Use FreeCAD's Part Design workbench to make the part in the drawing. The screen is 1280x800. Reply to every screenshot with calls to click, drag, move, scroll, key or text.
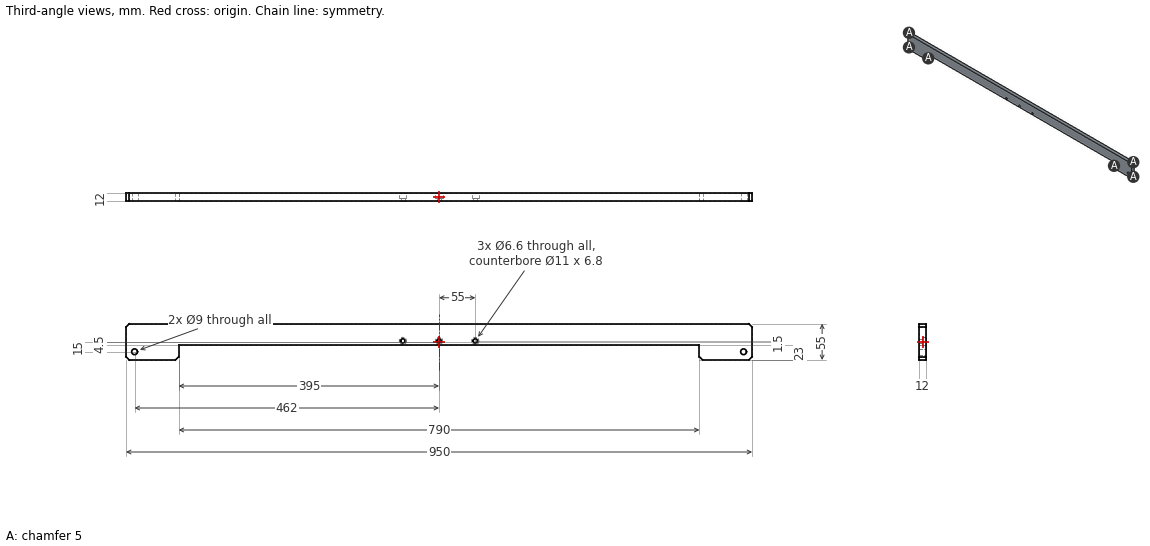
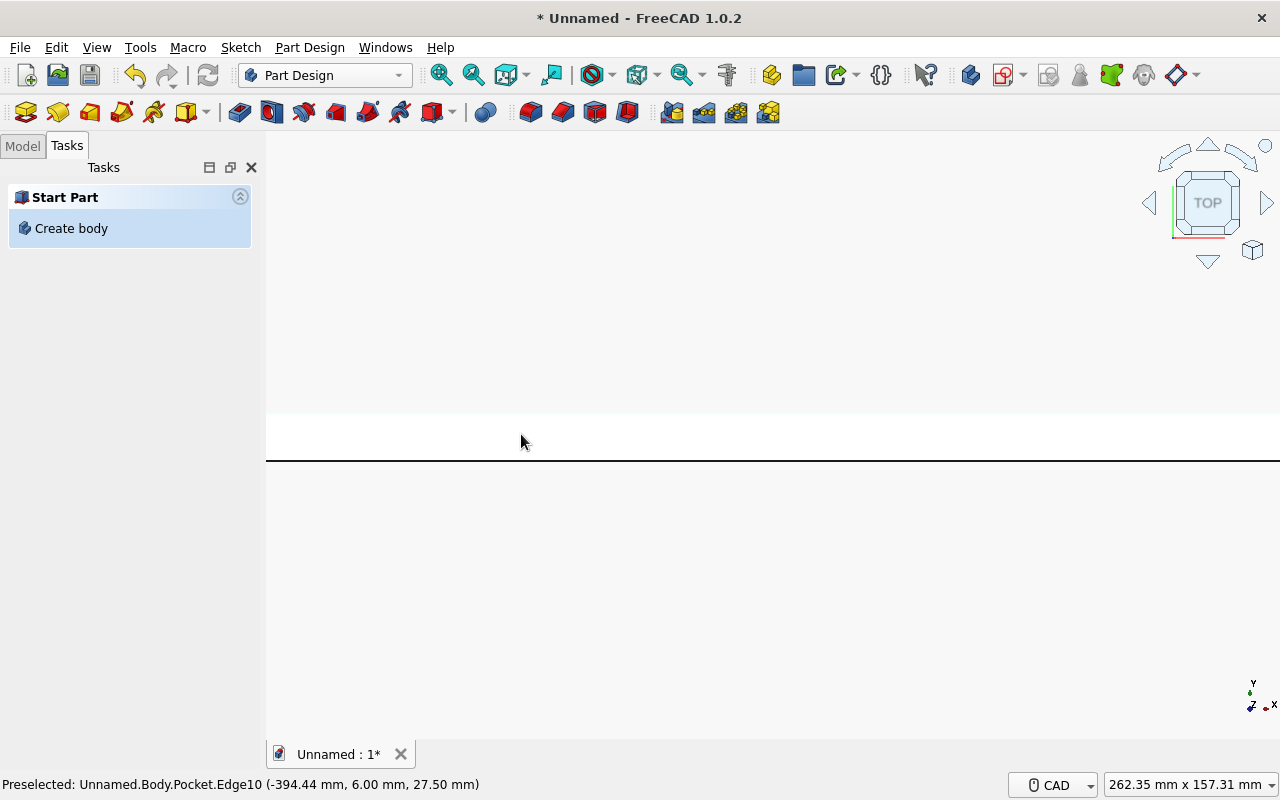
key(v)
key(f)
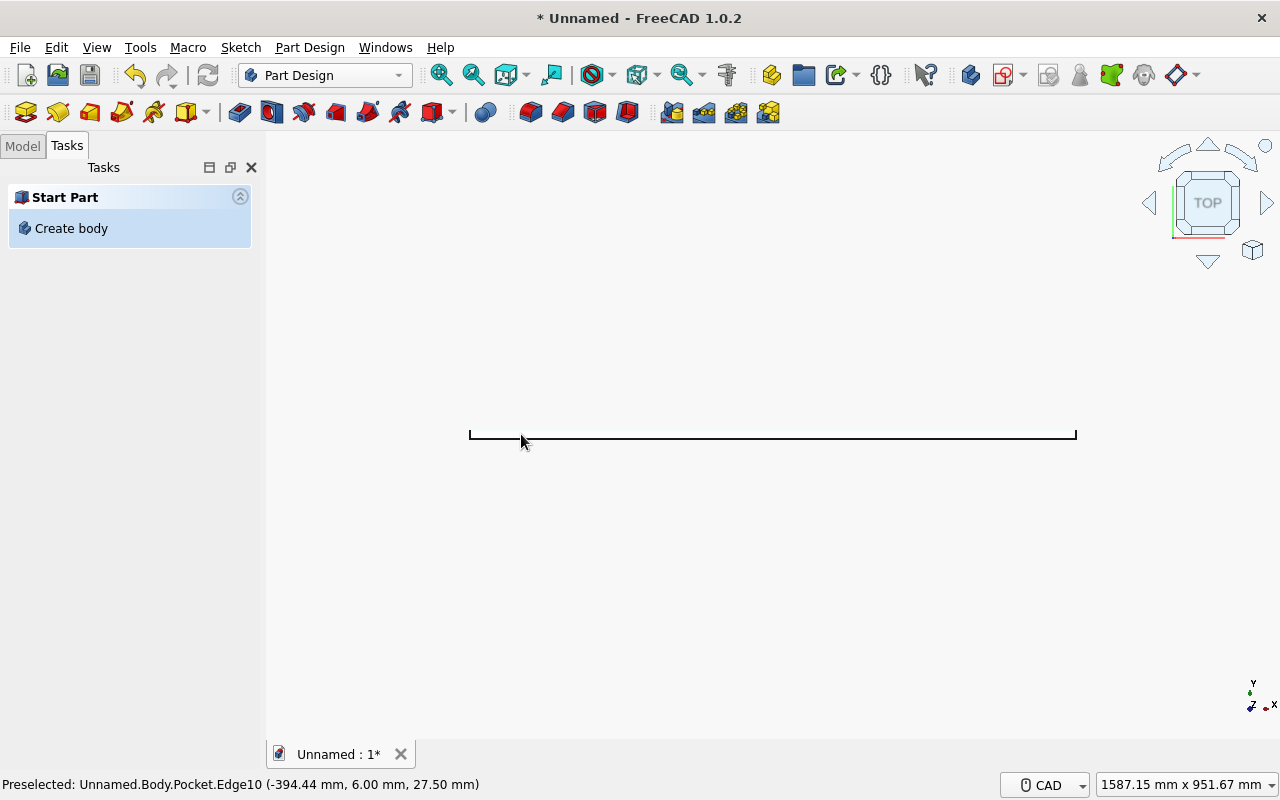
key(1)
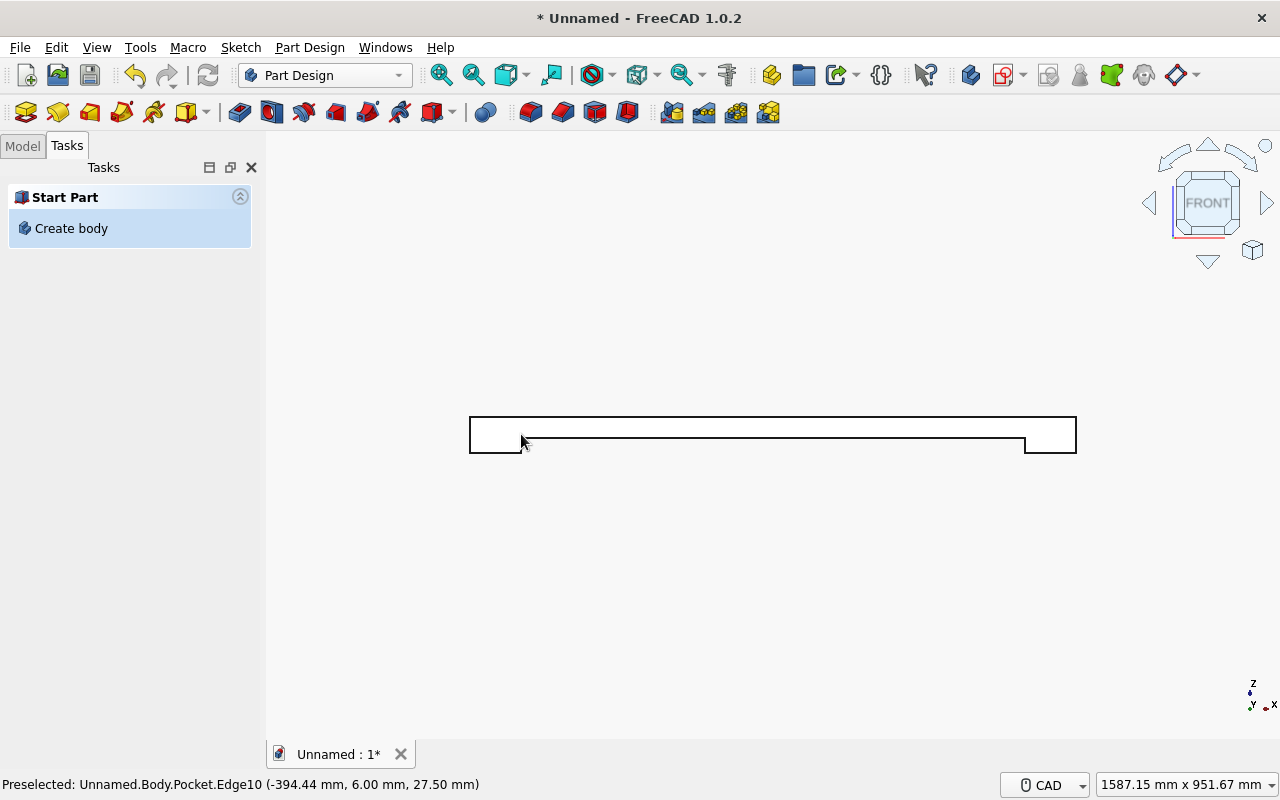
scroll(521, 452, up, 9)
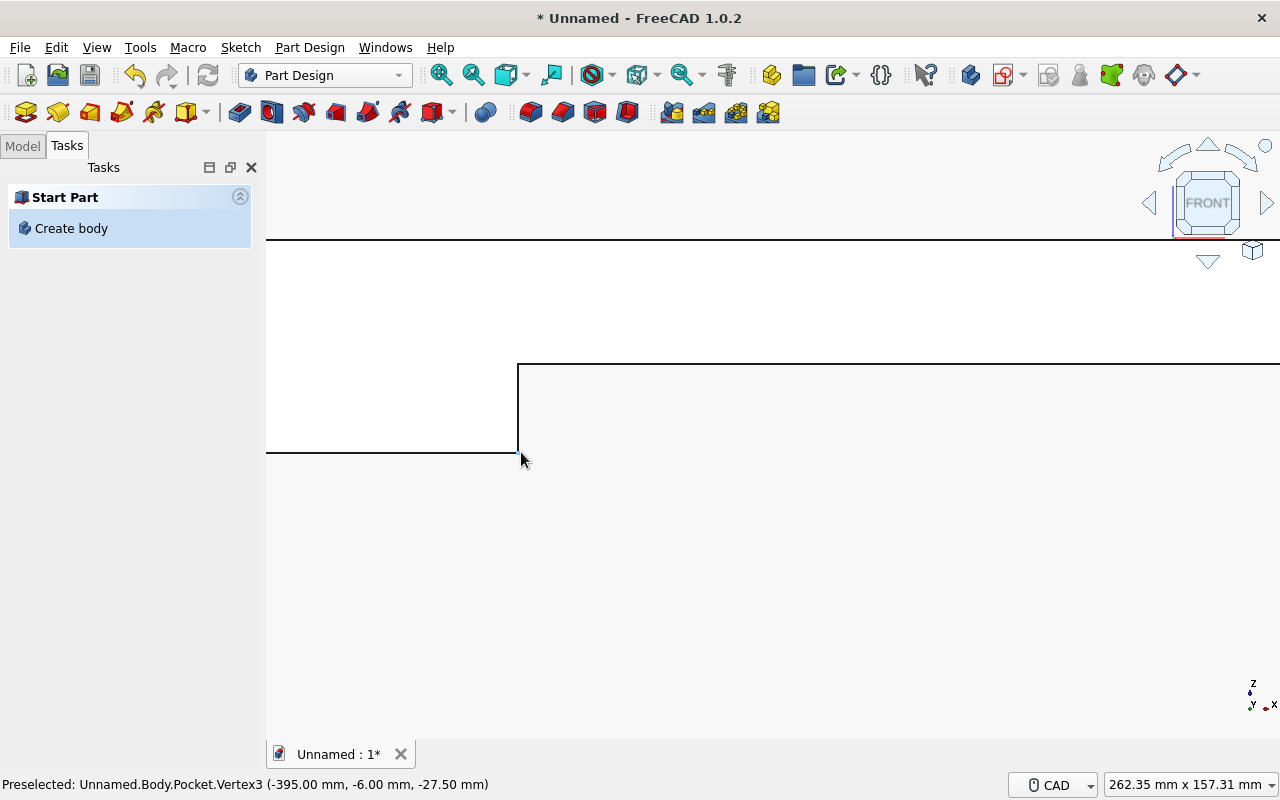
key(v)
key(f)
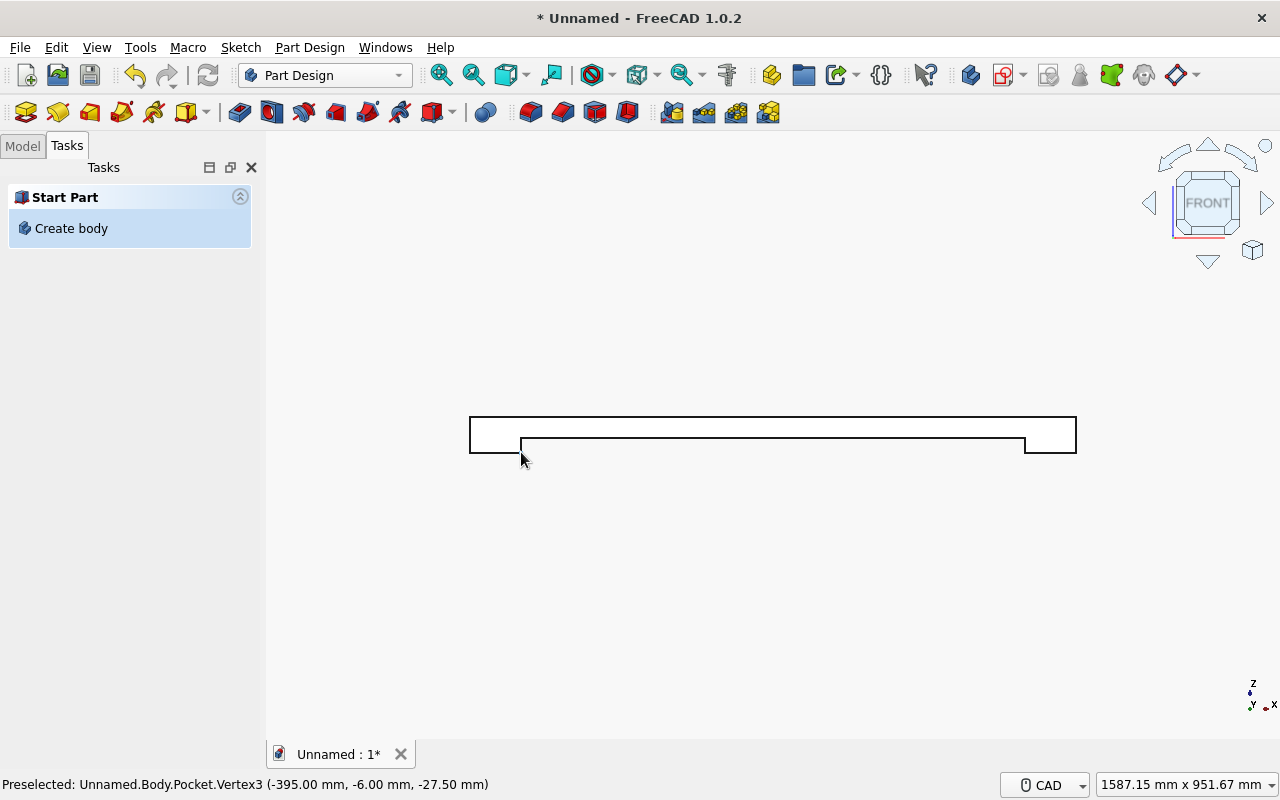
key(3)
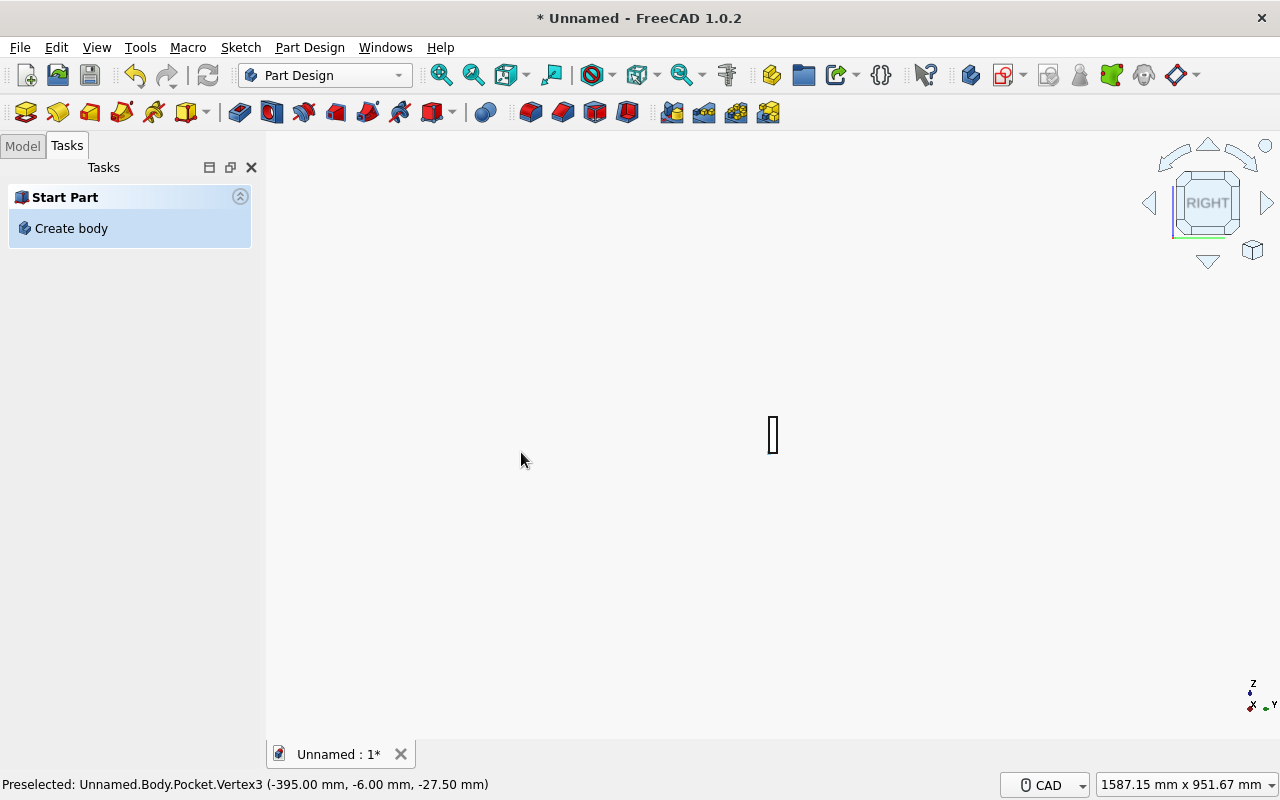
key(v)
key(f)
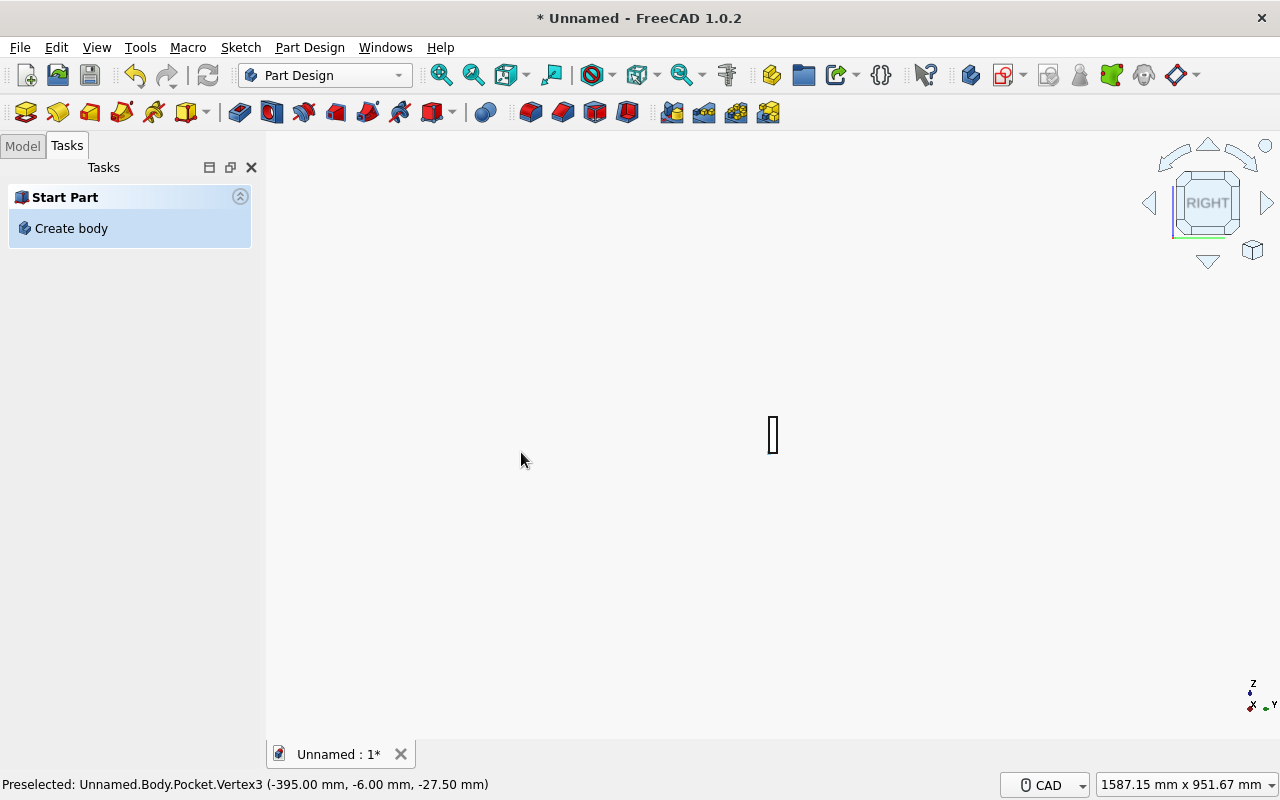
scroll(773, 452, up, 9)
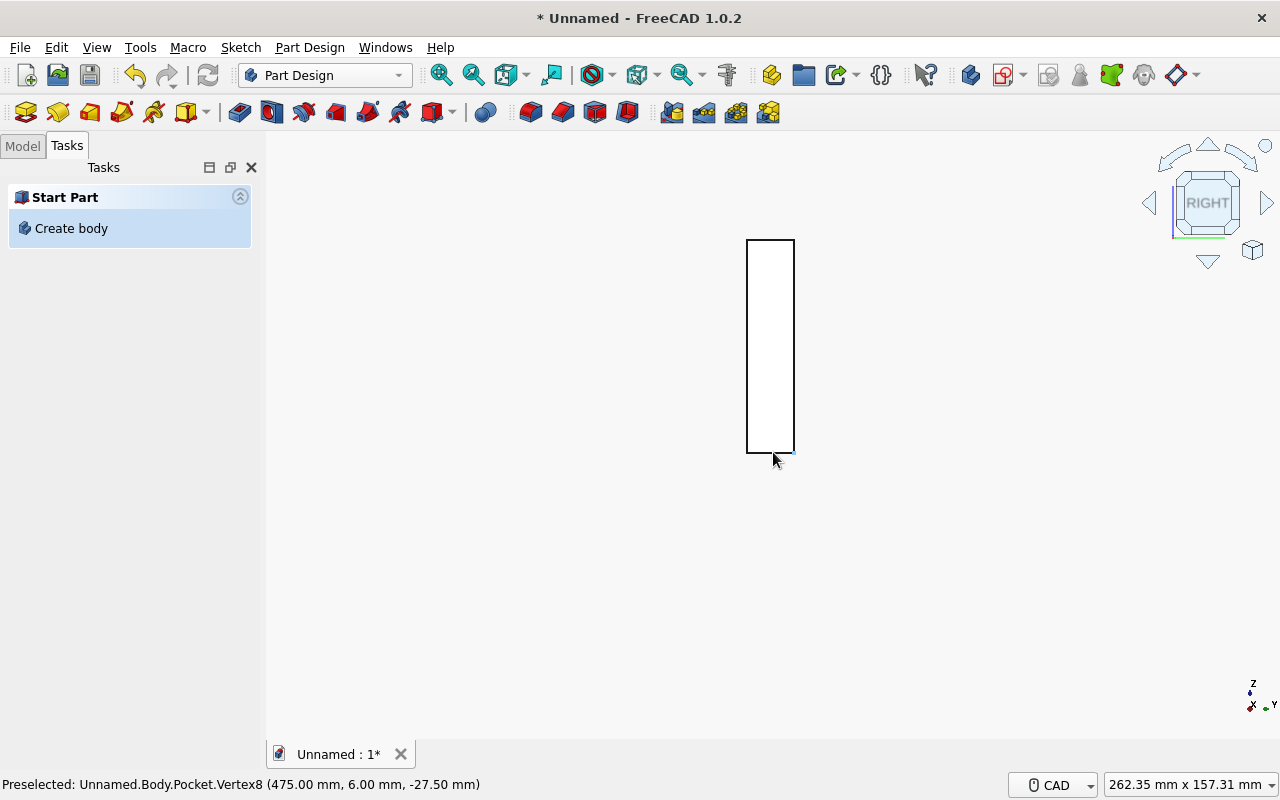
click(770, 239)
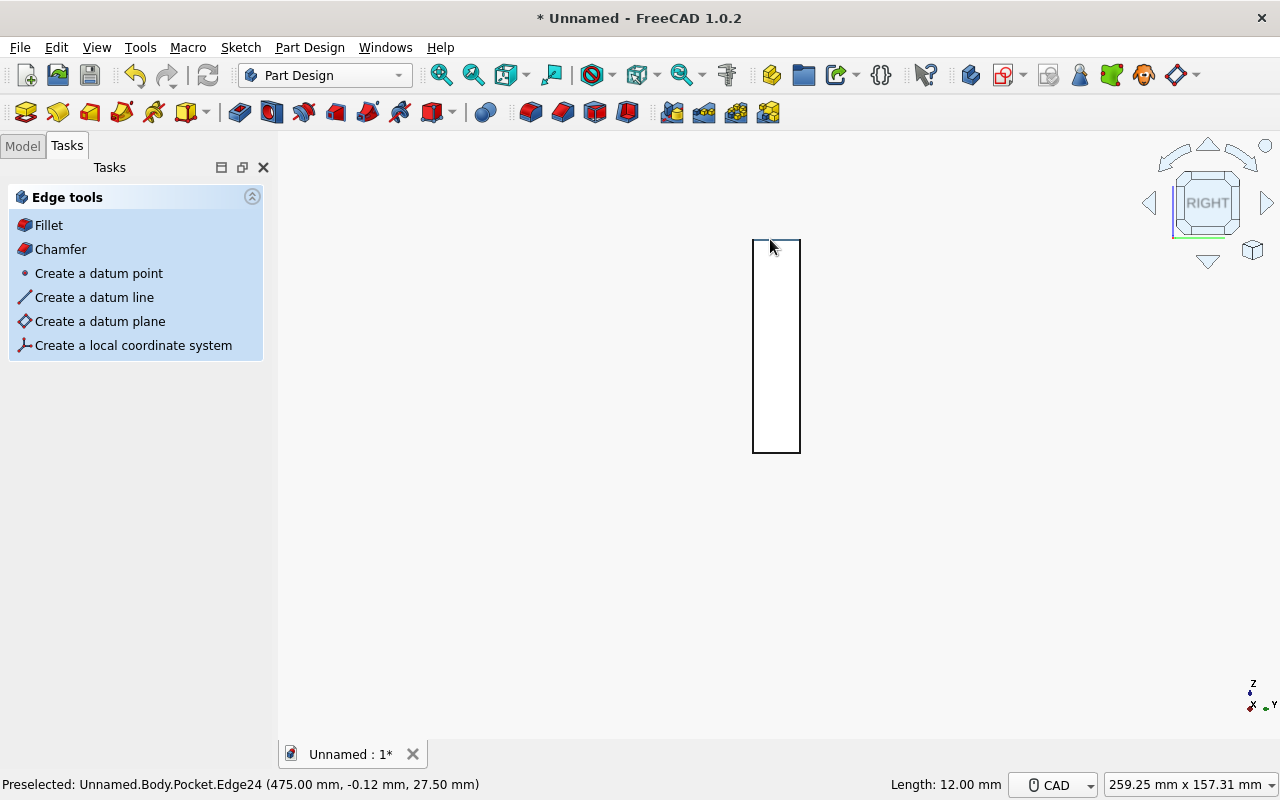
click(776, 452, ctrl)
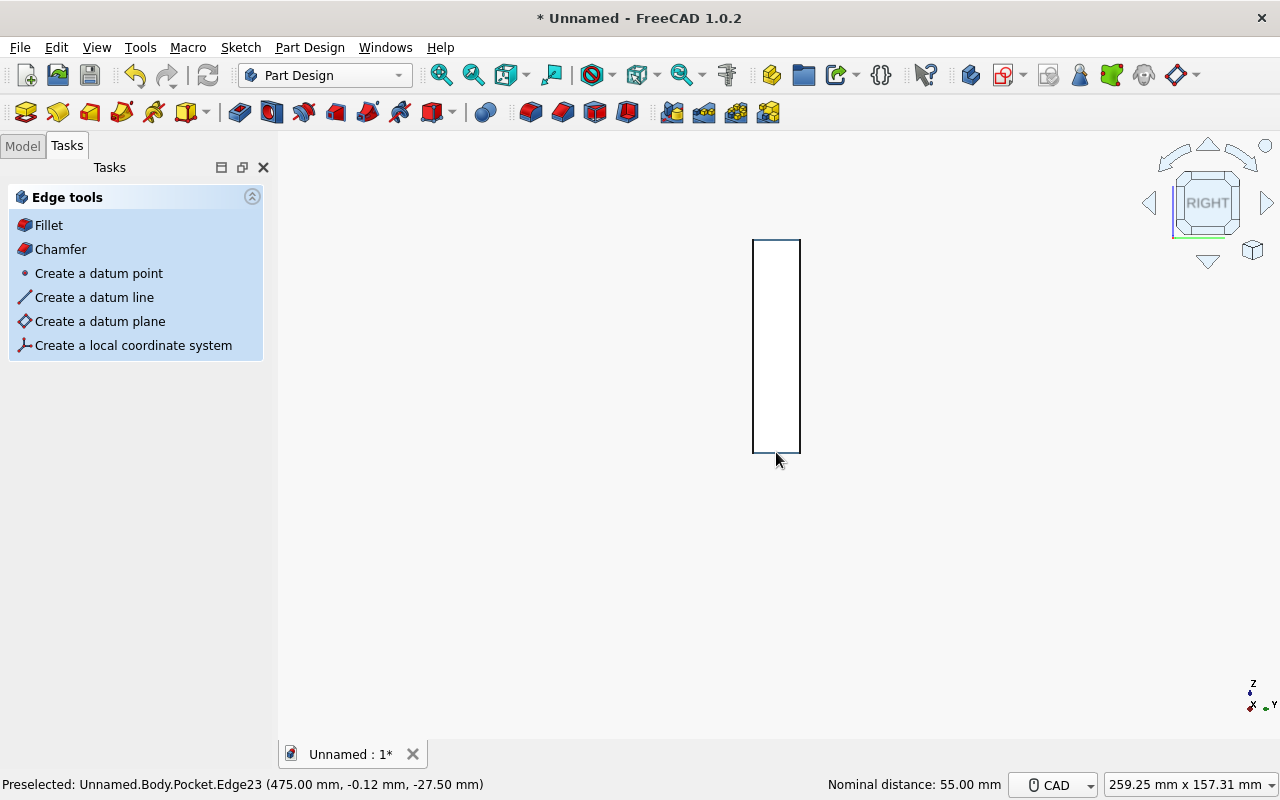
key(v)
key(f)